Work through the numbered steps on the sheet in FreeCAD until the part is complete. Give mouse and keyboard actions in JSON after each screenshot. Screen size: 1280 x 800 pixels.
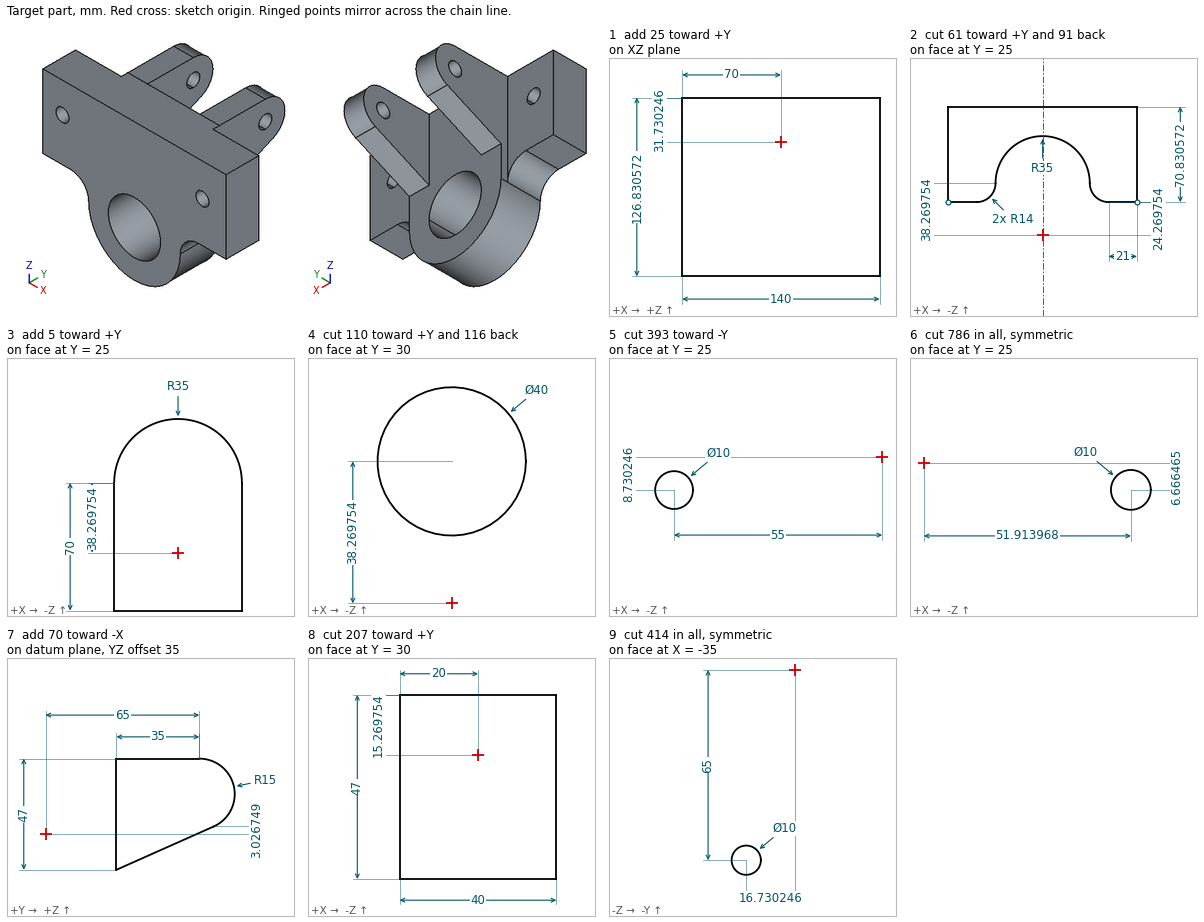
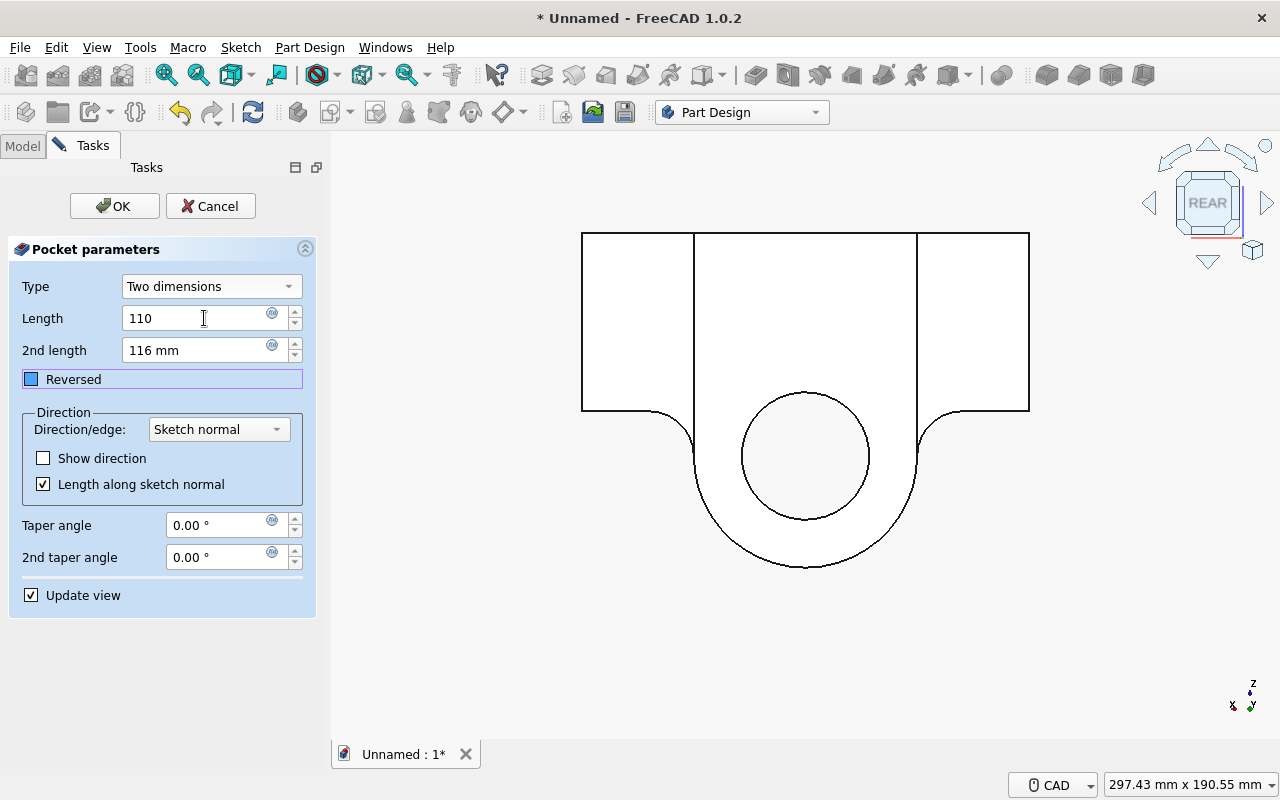
{"action": "left_click", "coordinate": [30, 379]}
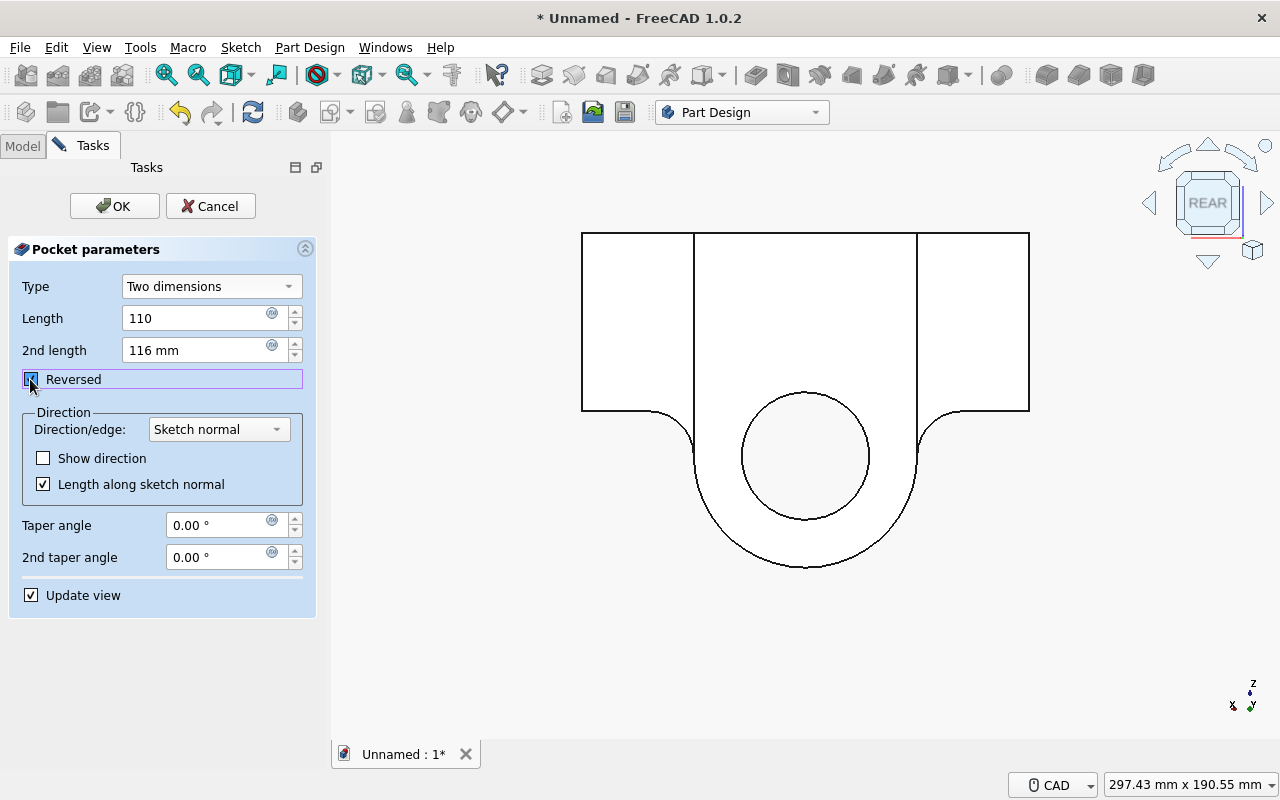
{"action": "left_click", "coordinate": [115, 206]}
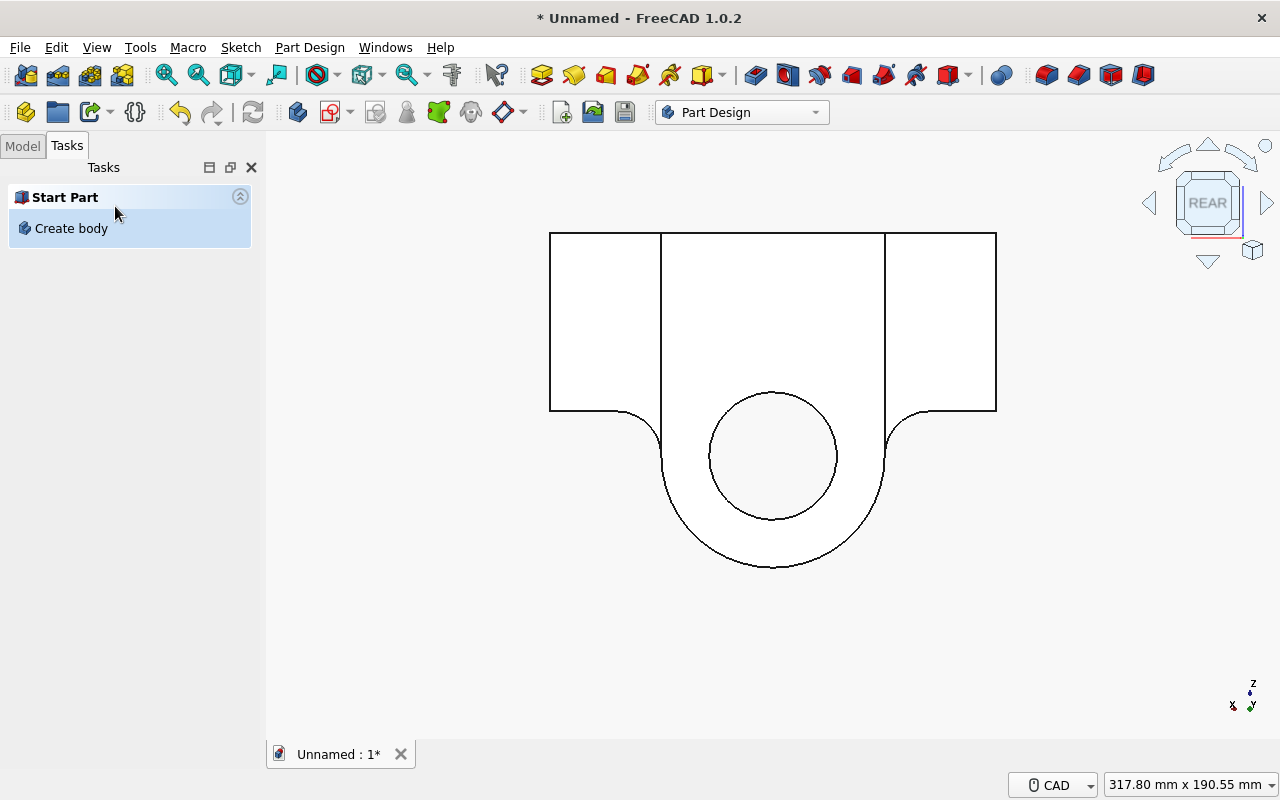
{"action": "left_click", "coordinate": [605, 311]}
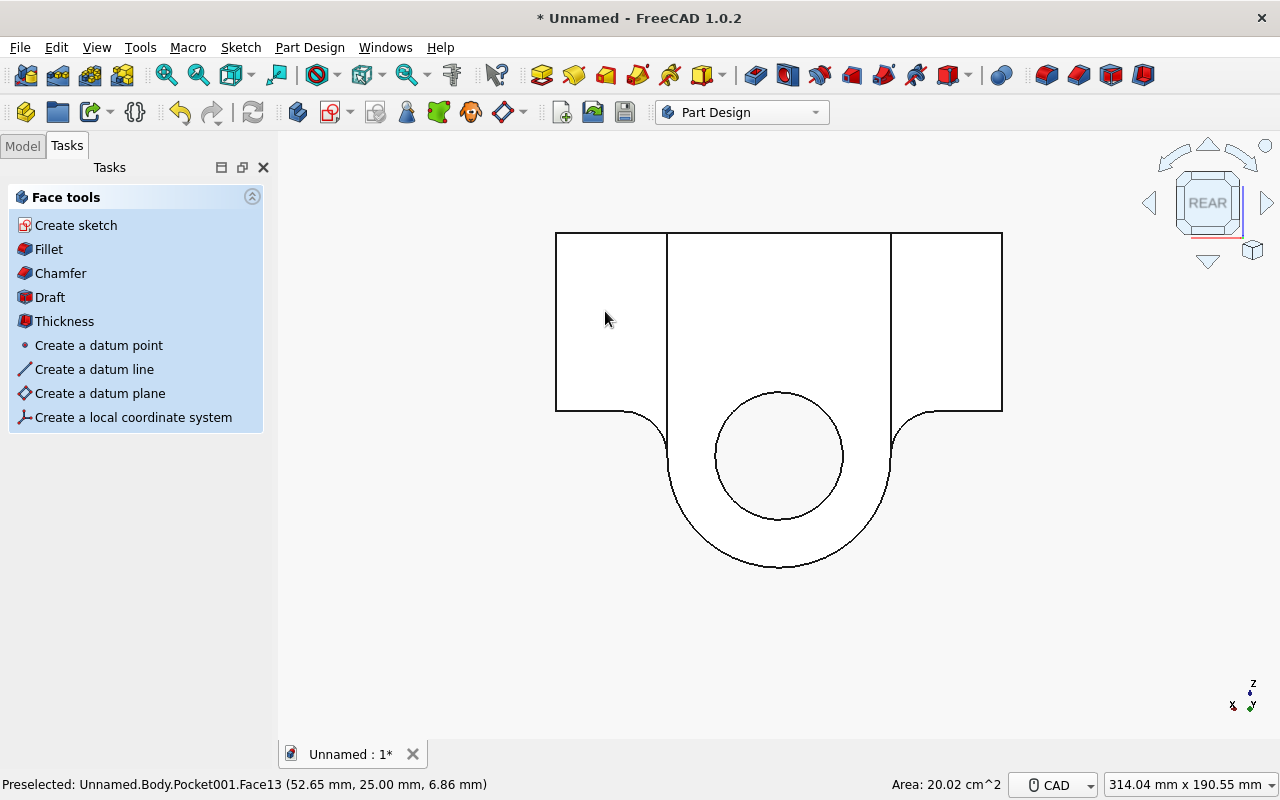
{"action": "left_click", "coordinate": [330, 112]}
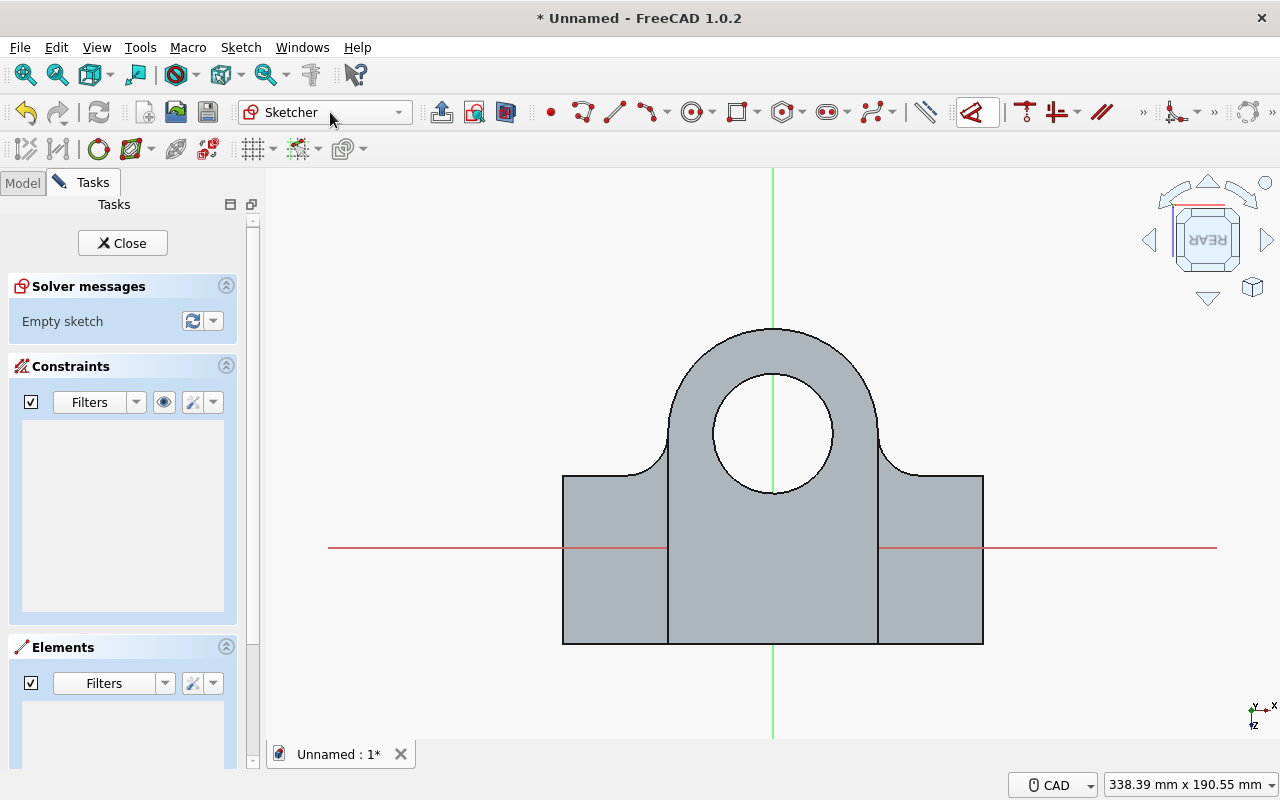
{"action": "left_click", "coordinate": [506, 112]}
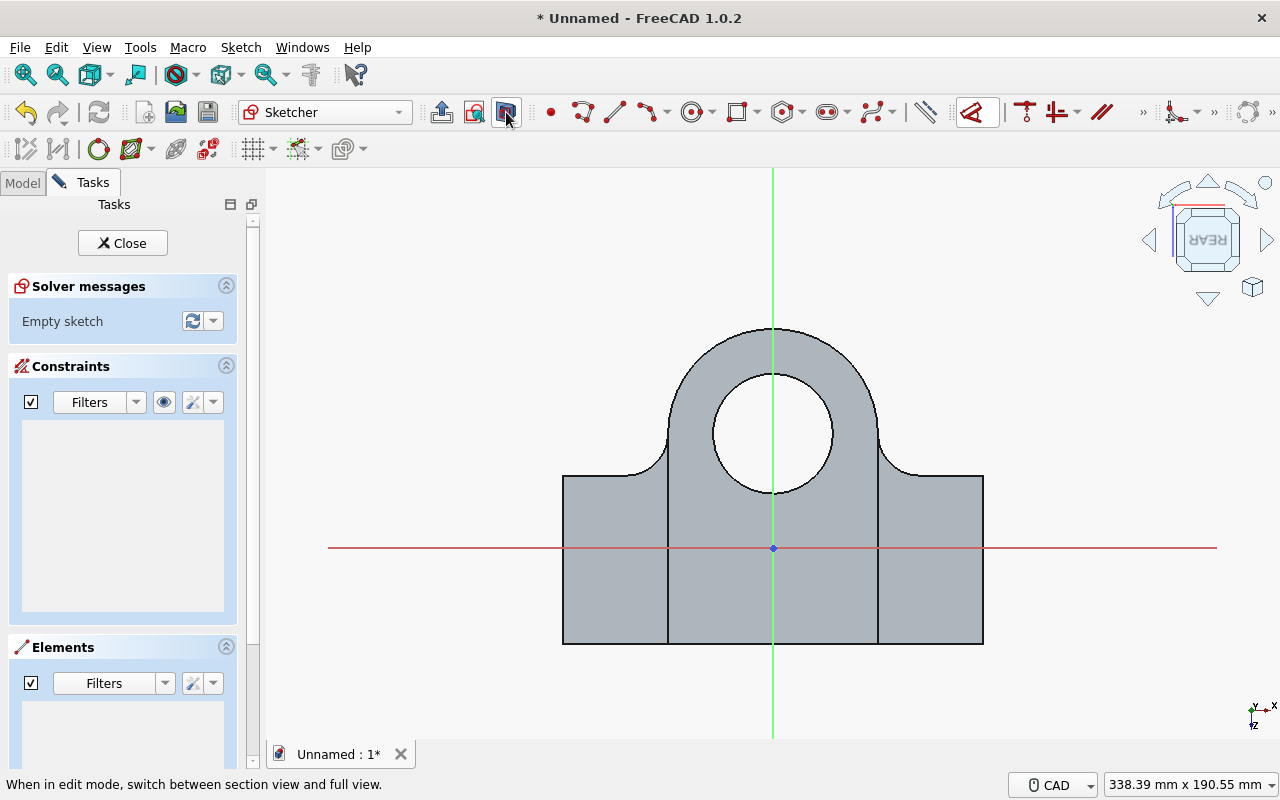
{"action": "scroll", "coordinate": [599, 587], "scroll_direction": "up", "scroll_amount": 12}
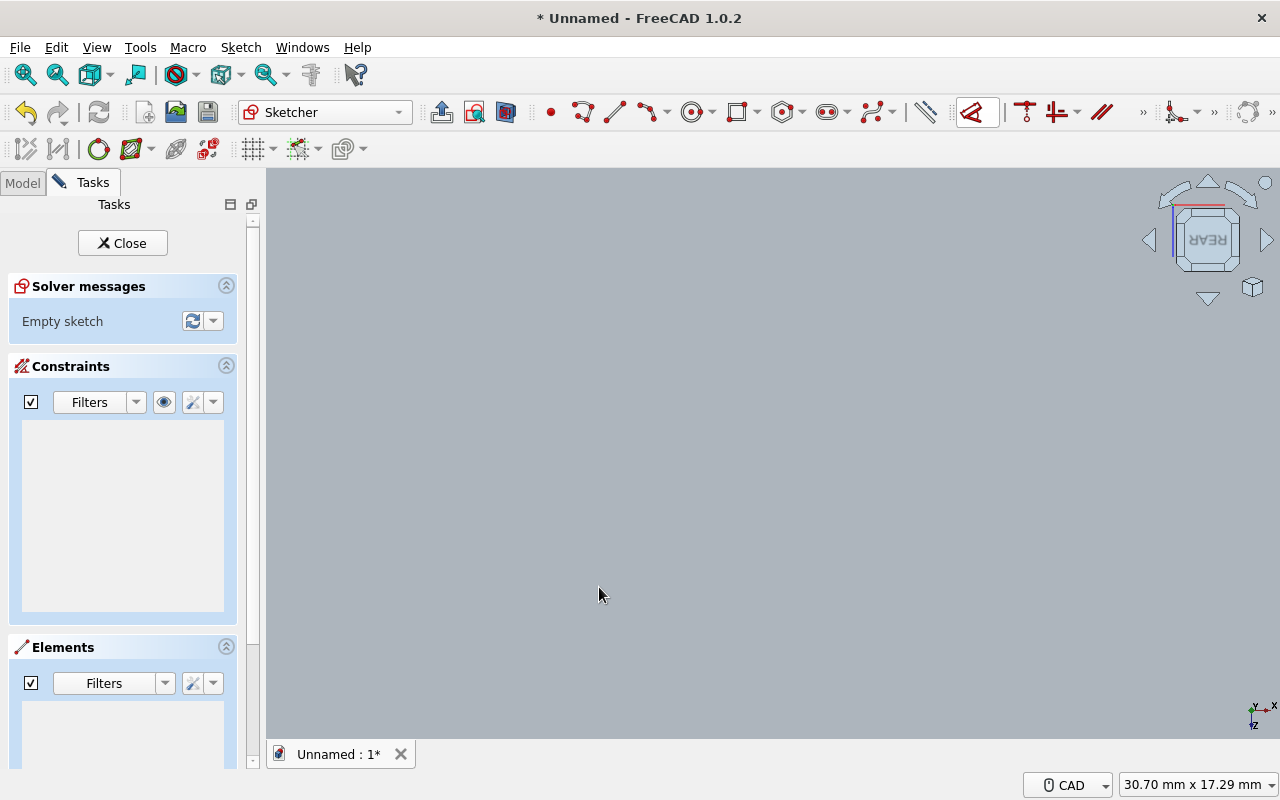
{"action": "left_click", "coordinate": [692, 112]}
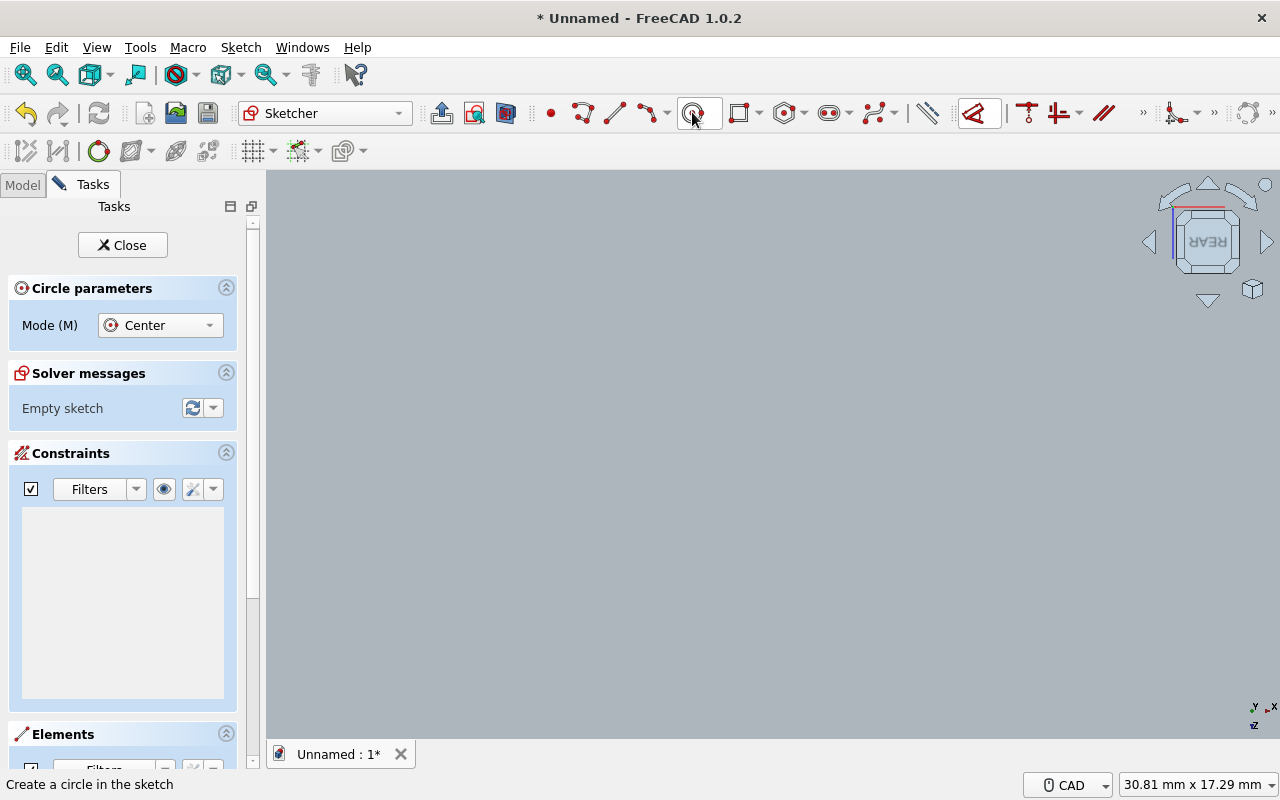
{"action": "left_click", "coordinate": [697, 444]}
{"action": "left_click", "coordinate": [814, 328]}
{"action": "key", "text": "Escape"}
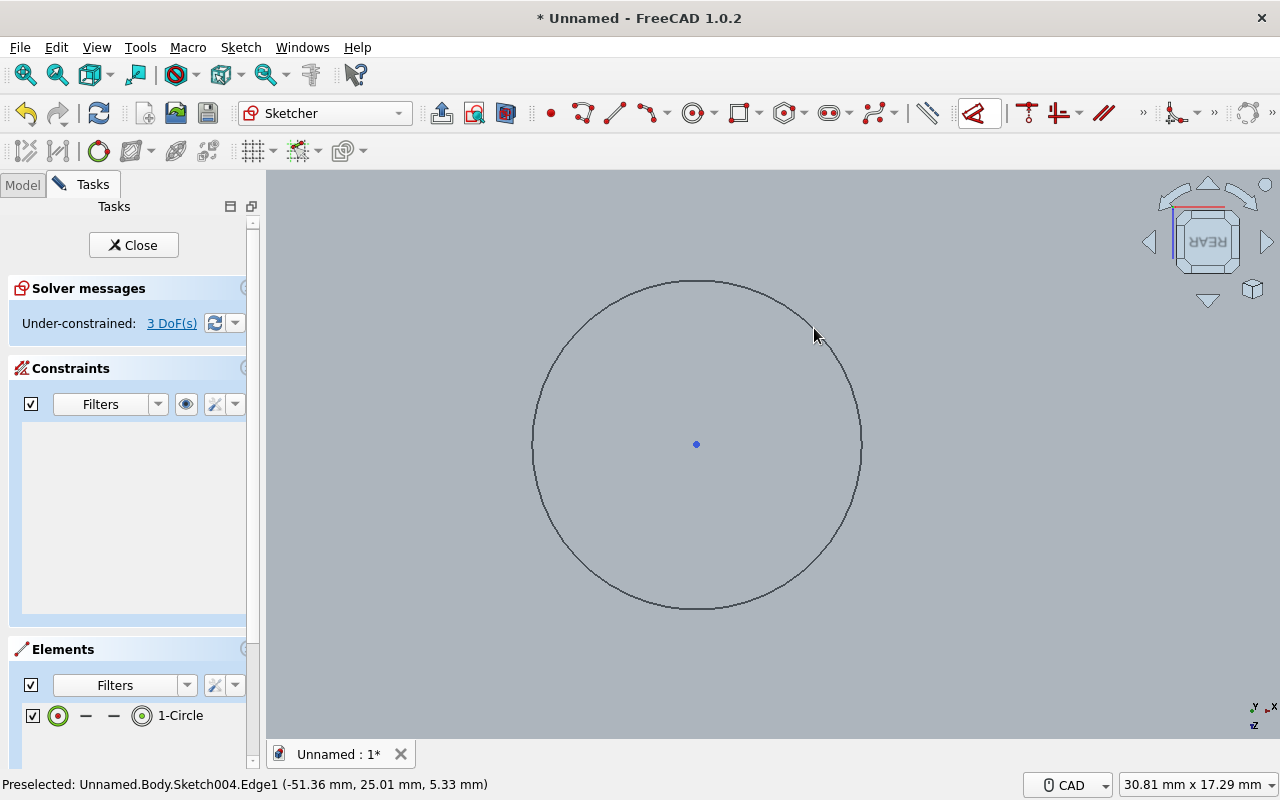
{"action": "left_click", "coordinate": [813, 328]}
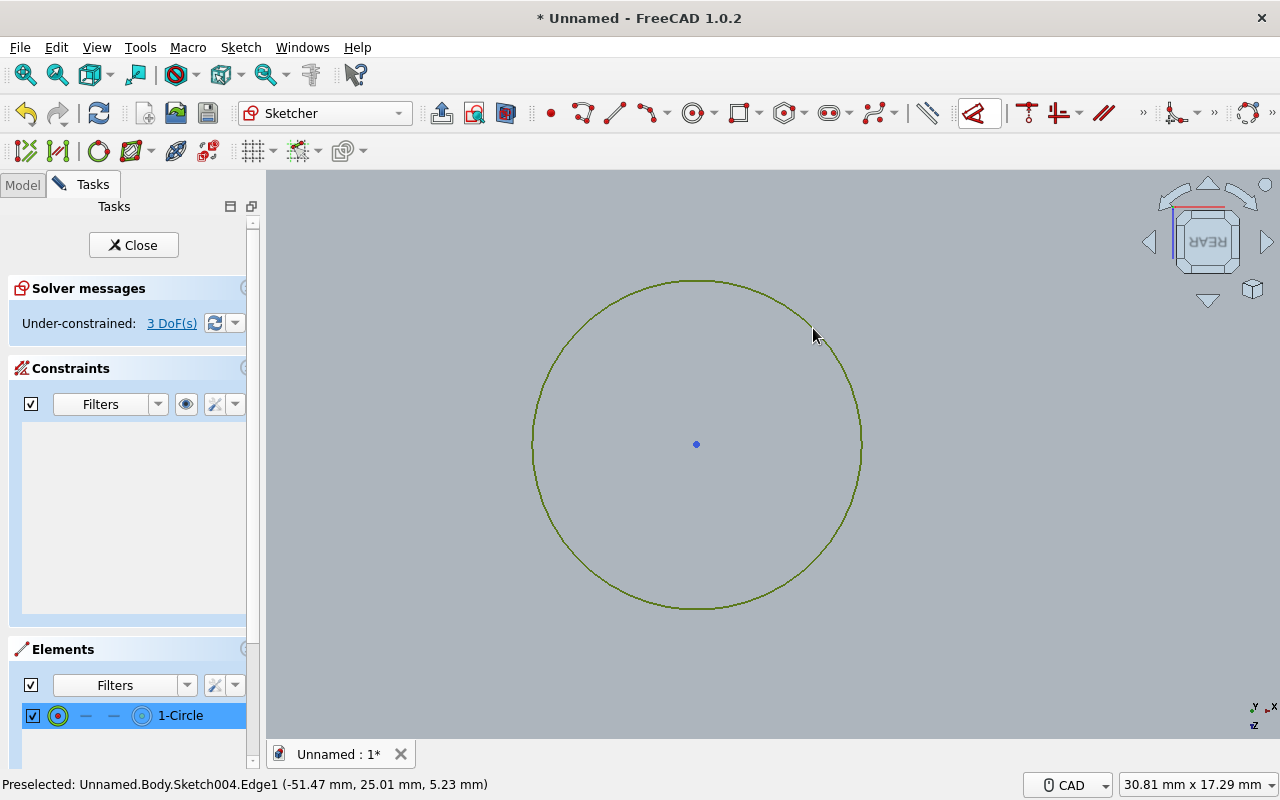
{"action": "left_click", "coordinate": [996, 114]}